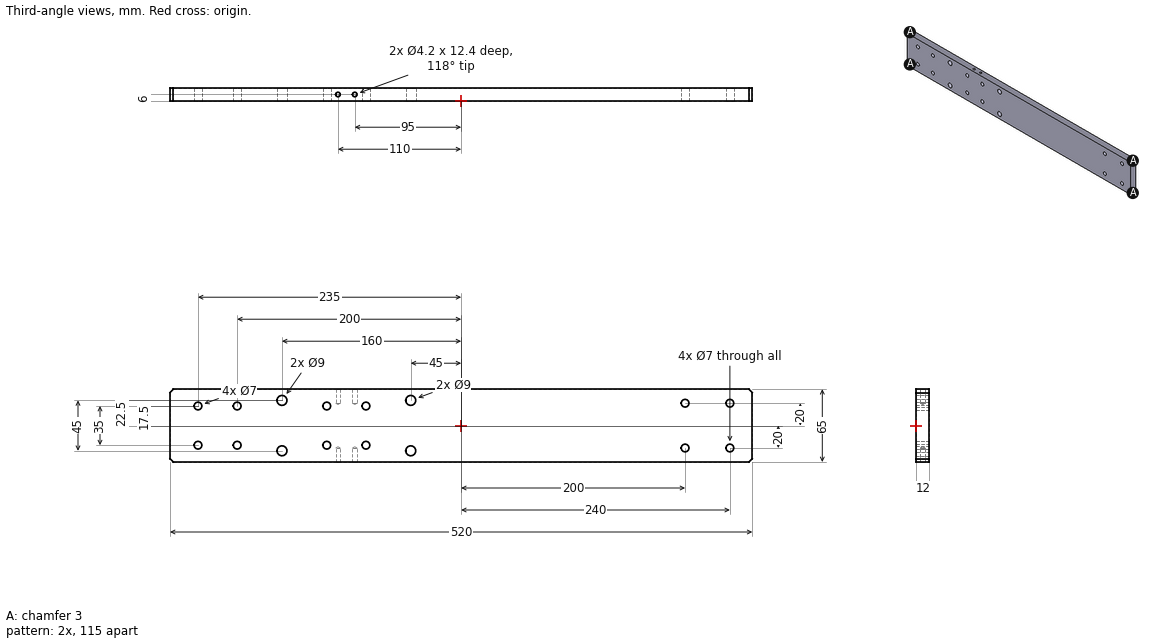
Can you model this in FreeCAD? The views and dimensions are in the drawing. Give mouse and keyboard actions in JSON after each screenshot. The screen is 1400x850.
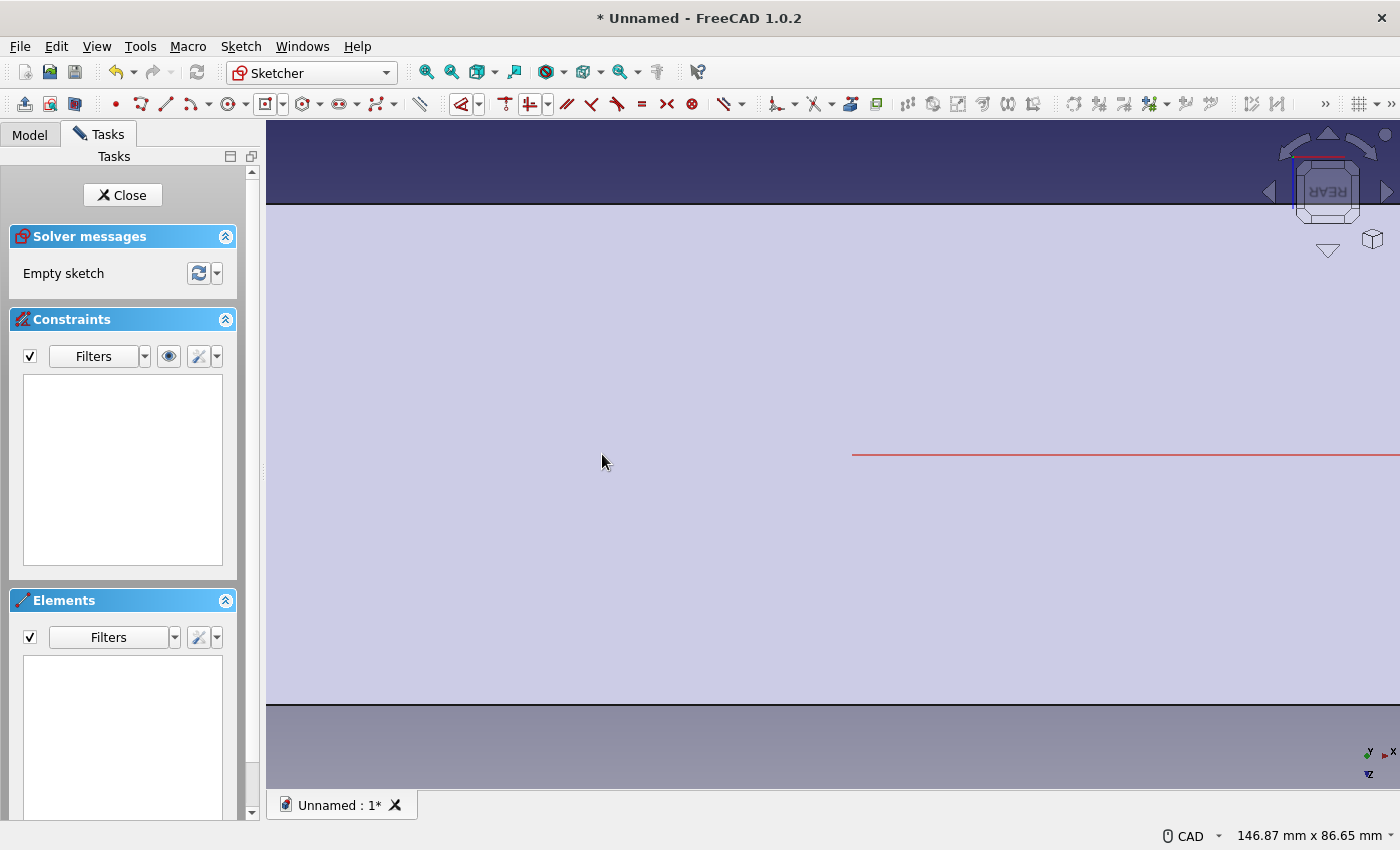
{"action": "left_click", "coordinate": [228, 104]}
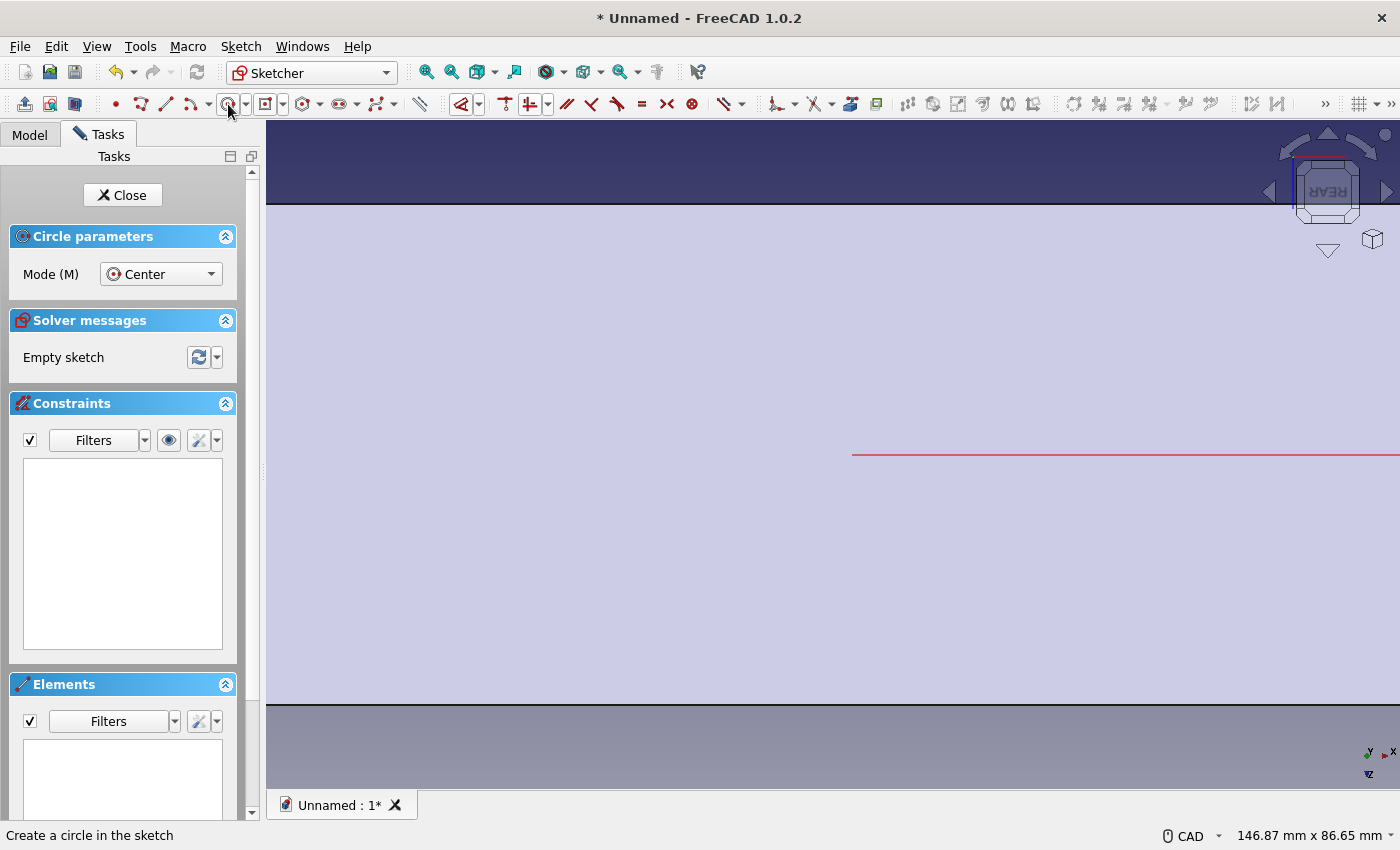
{"action": "left_click", "coordinate": [763, 628]}
{"action": "left_click", "coordinate": [787, 604]}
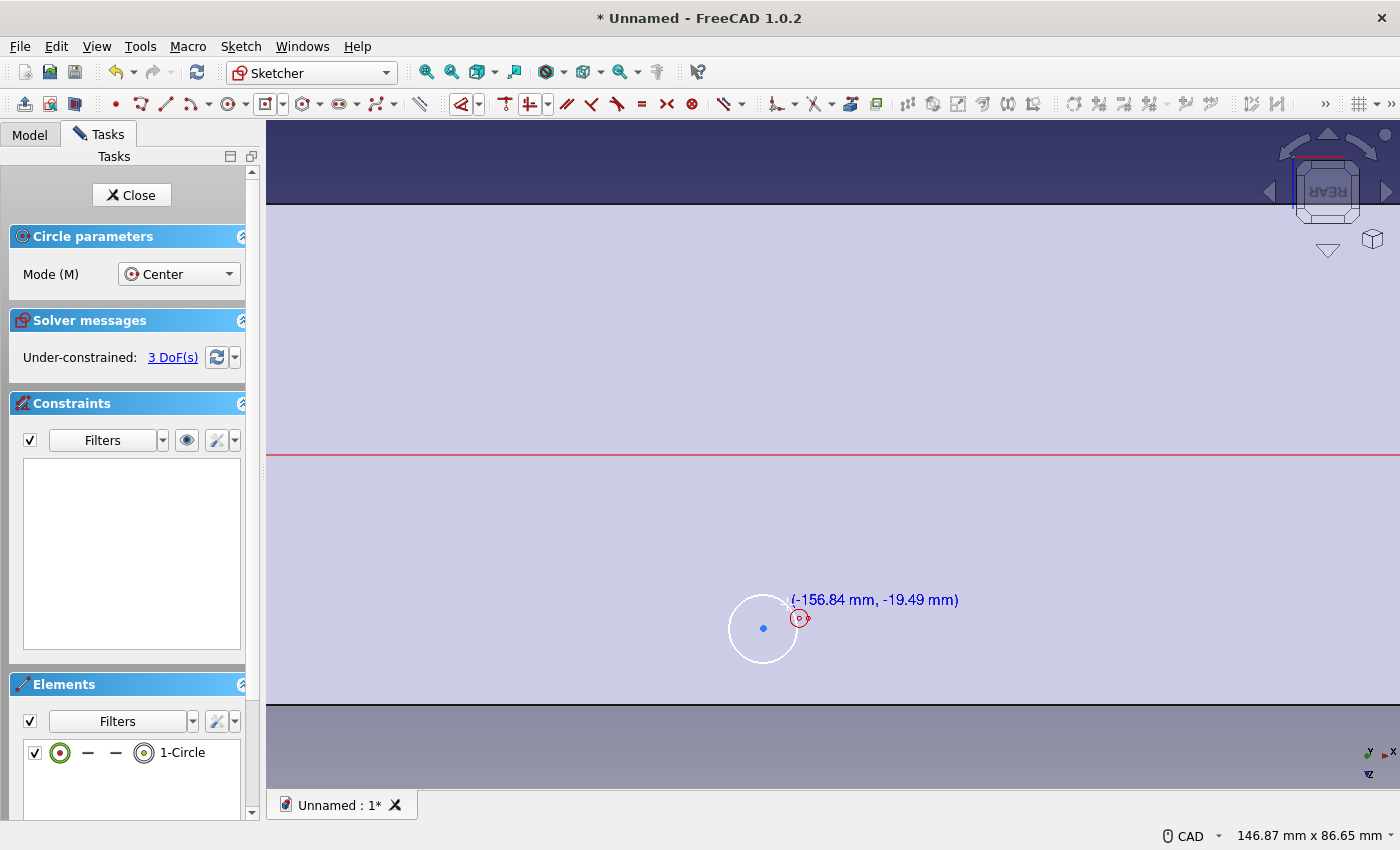
{"action": "left_click", "coordinate": [763, 281]}
{"action": "left_click", "coordinate": [787, 256]}
{"action": "key", "text": "Escape"}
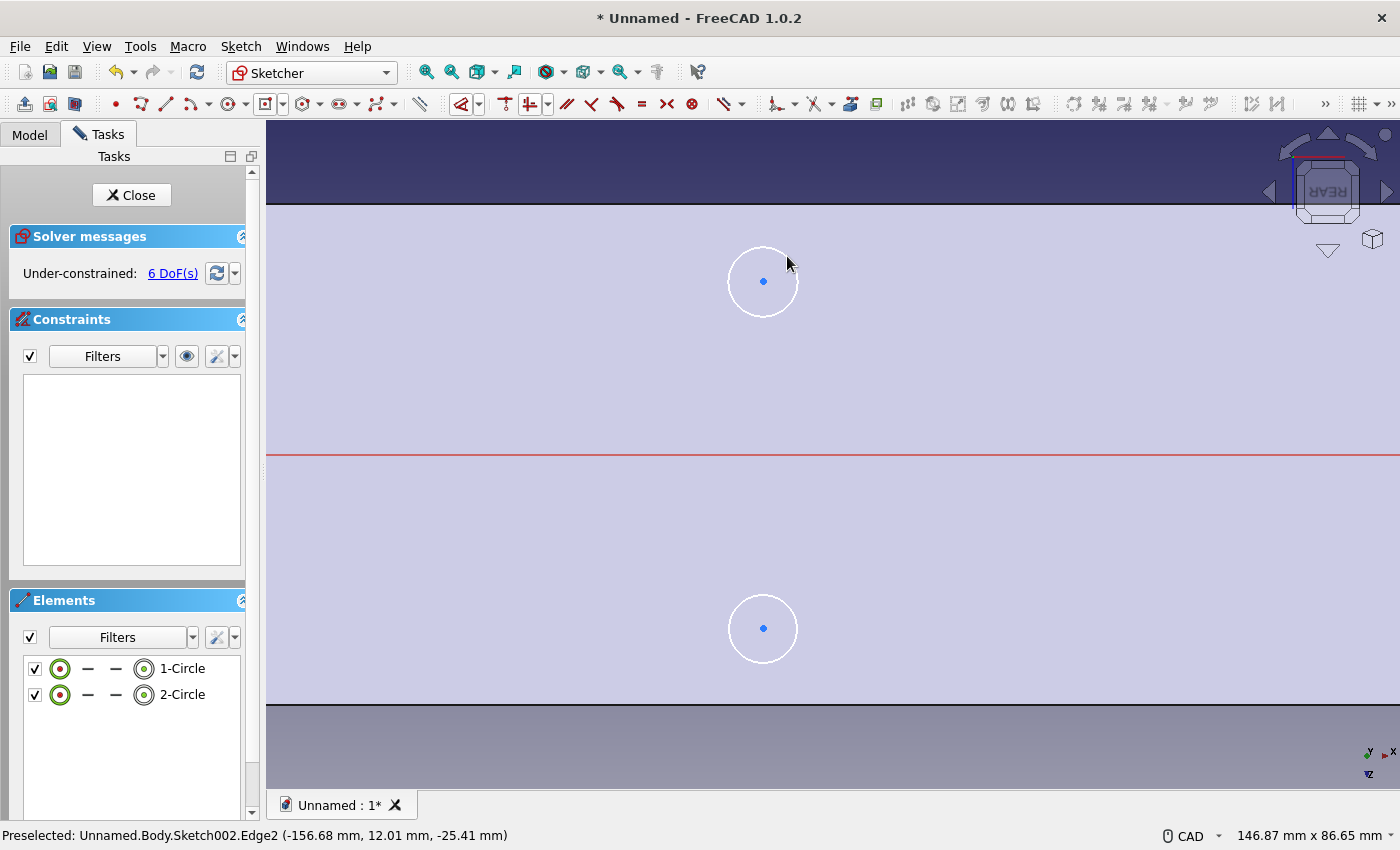
{"action": "left_click", "coordinate": [787, 605]}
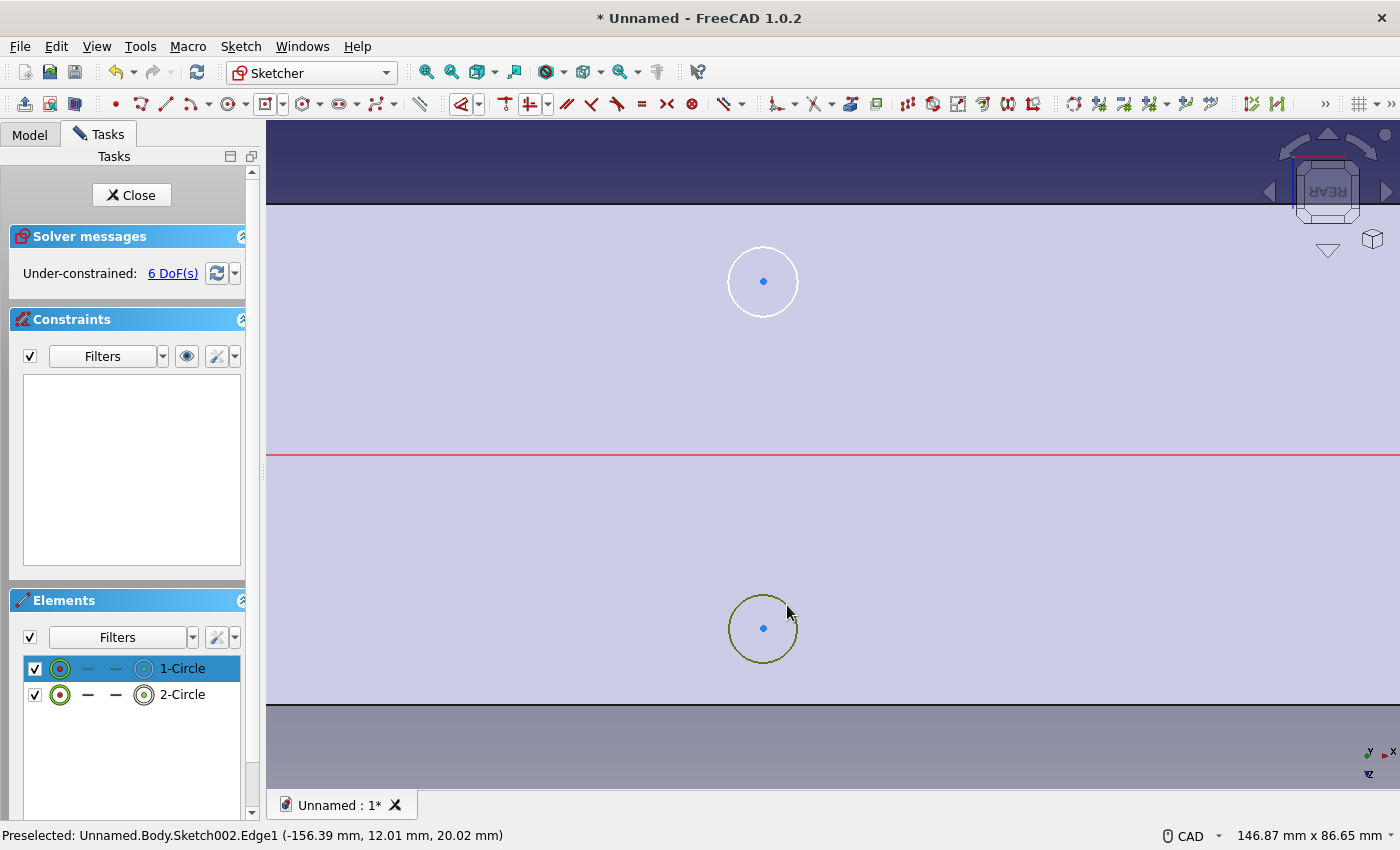
{"action": "left_click", "coordinate": [787, 257]}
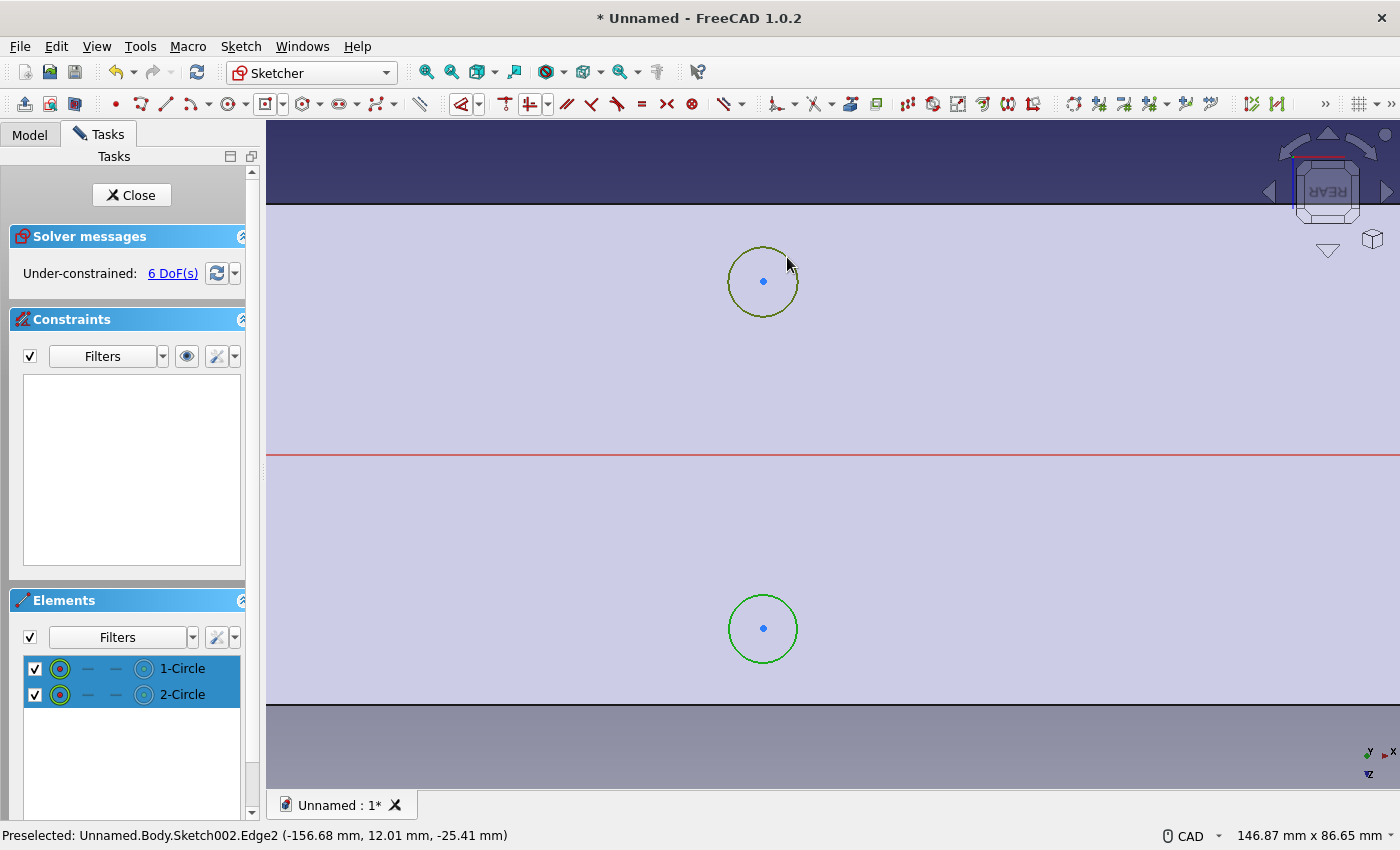
{"action": "left_click", "coordinate": [642, 104]}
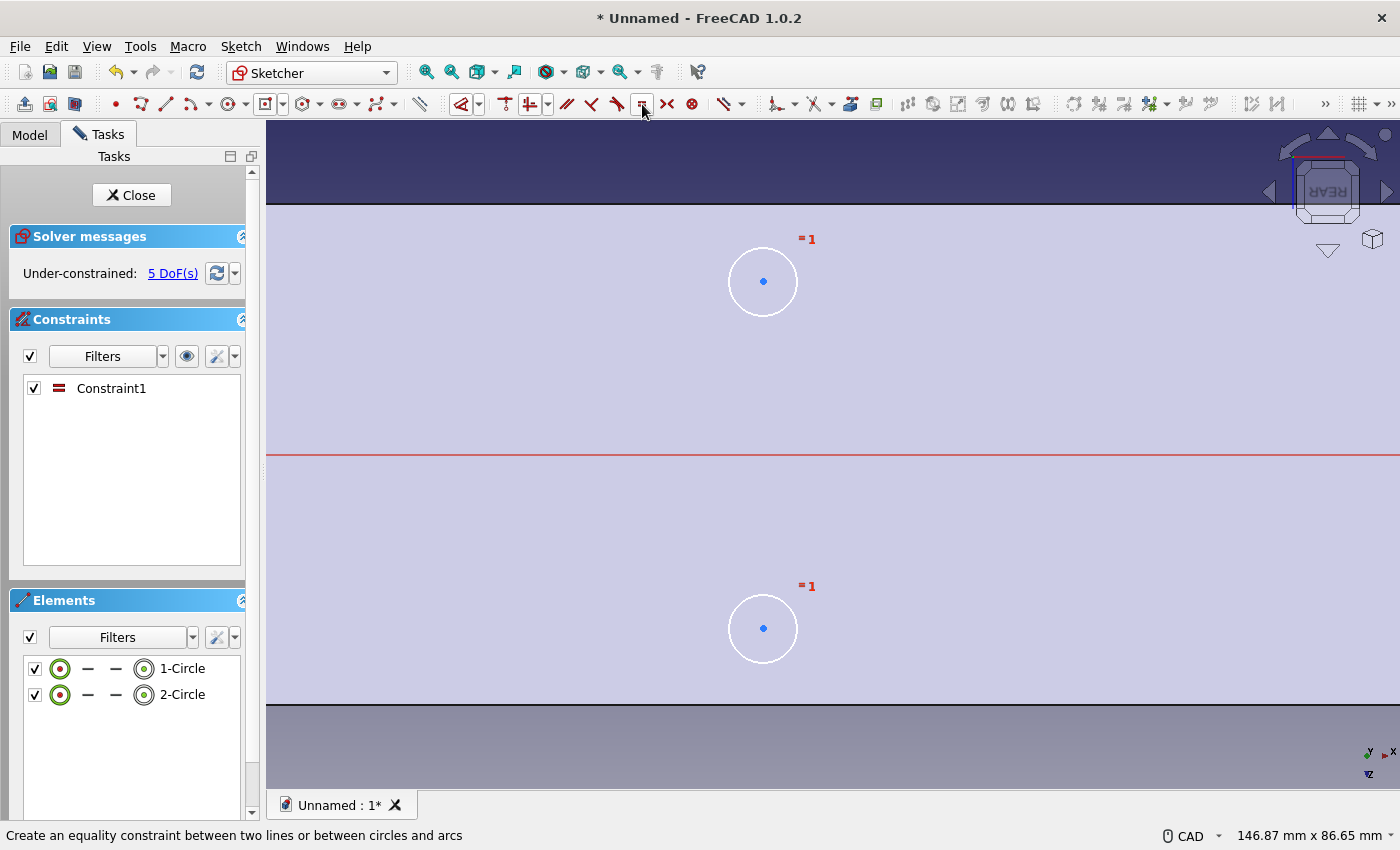
{"action": "left_click", "coordinate": [763, 629]}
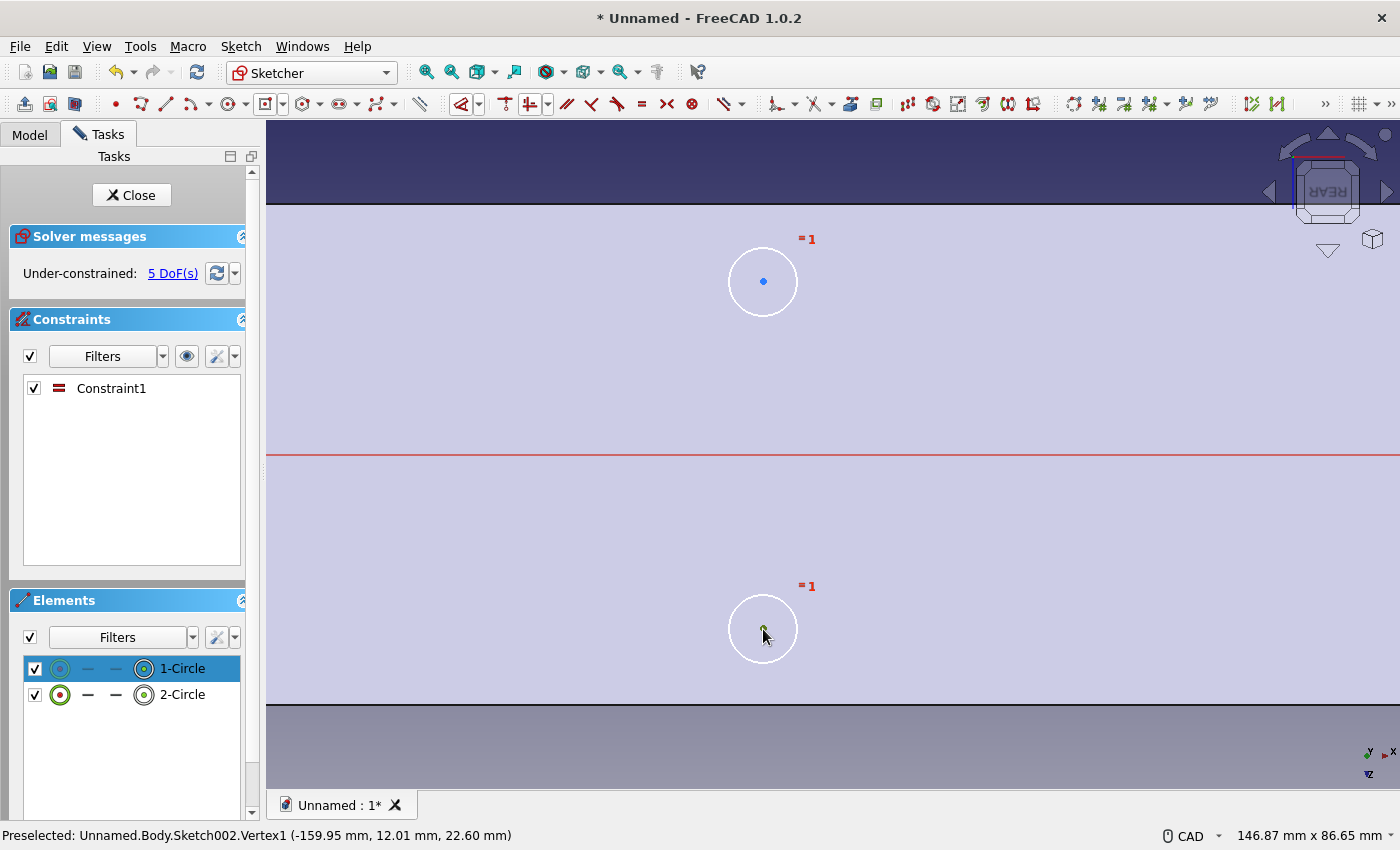
{"action": "left_click", "coordinate": [763, 282]}